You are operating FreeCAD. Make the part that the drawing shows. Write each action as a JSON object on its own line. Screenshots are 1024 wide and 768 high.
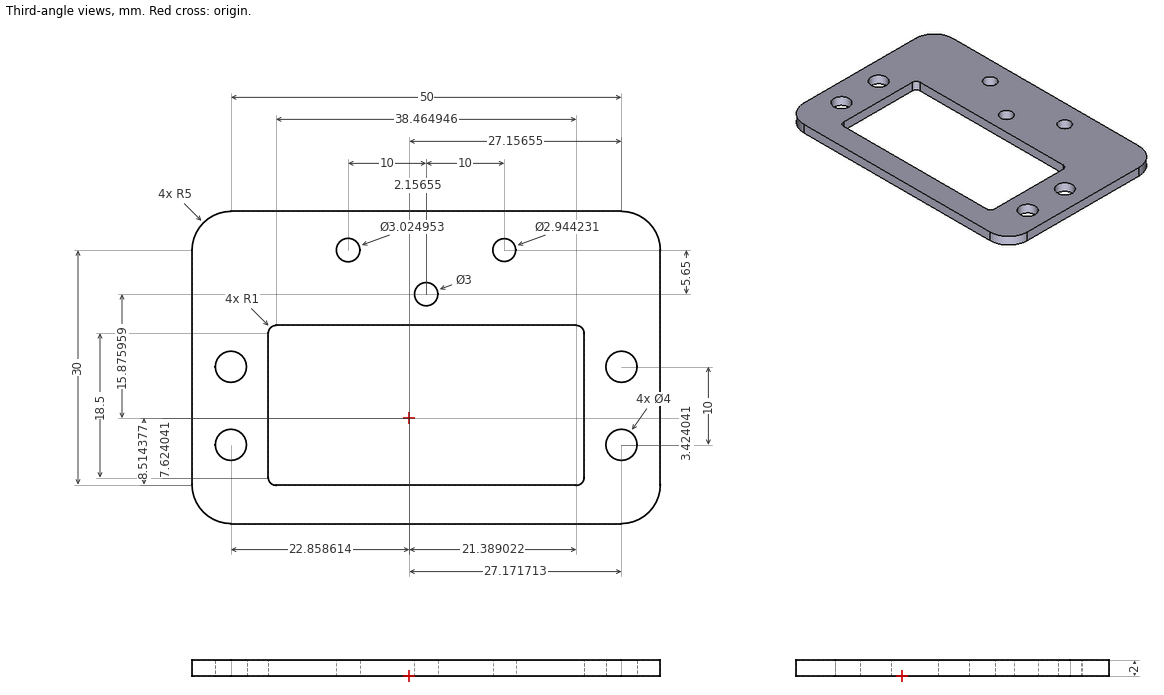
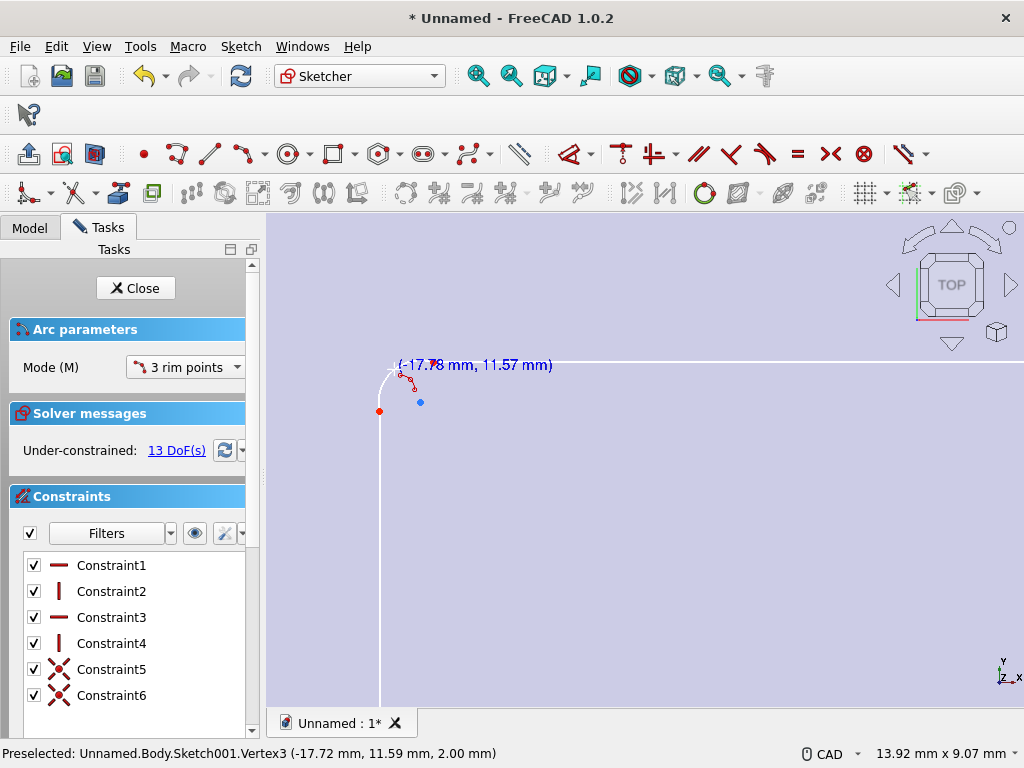
{"action": "scroll", "coordinate": [398, 371], "scroll_direction": "down", "scroll_amount": 9}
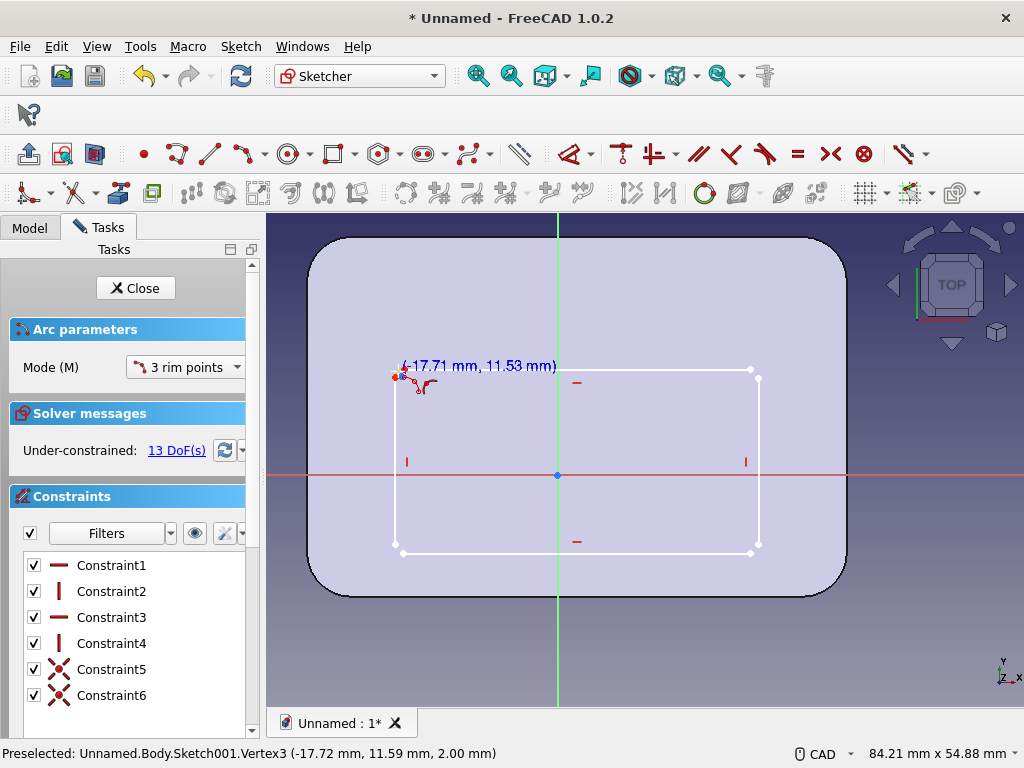
{"action": "scroll", "coordinate": [395, 544], "scroll_direction": "up", "scroll_amount": 2}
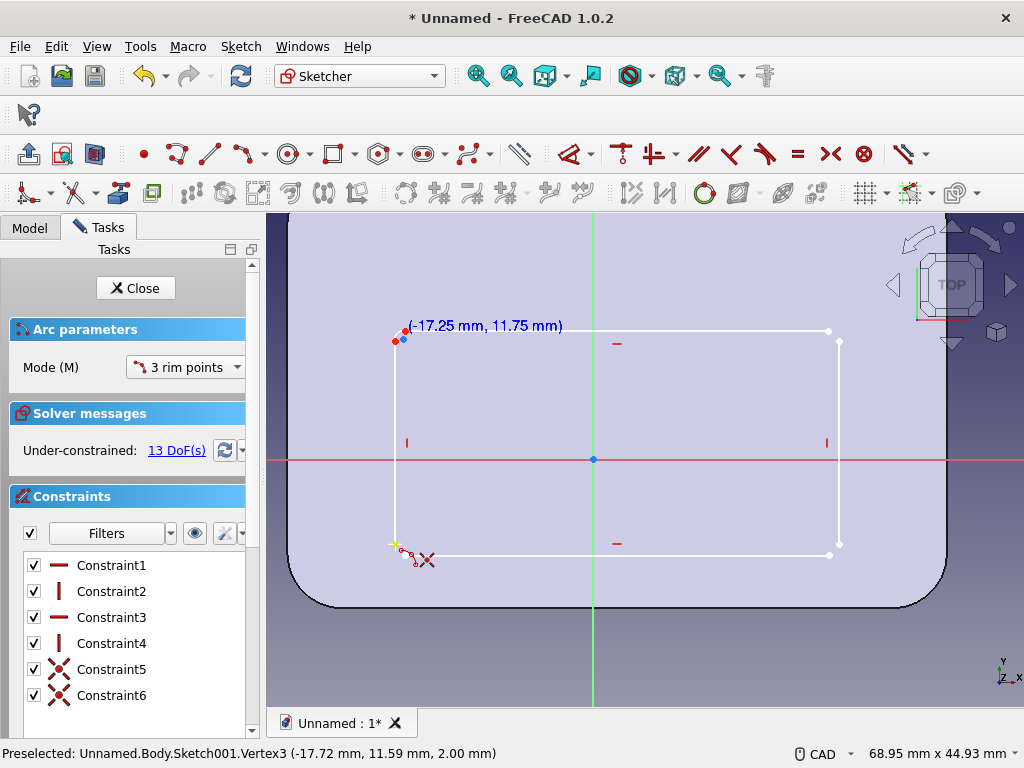
{"action": "left_click", "coordinate": [395, 545]}
{"action": "left_click", "coordinate": [408, 558]}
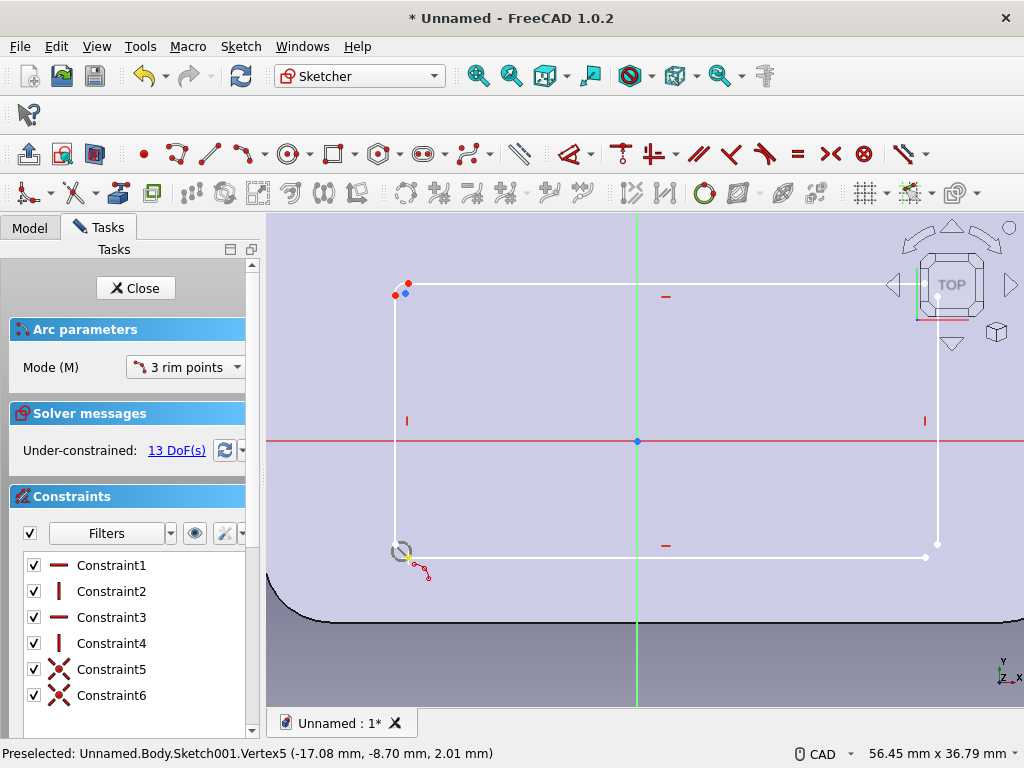
{"action": "scroll", "coordinate": [399, 553], "scroll_direction": "up", "scroll_amount": 7}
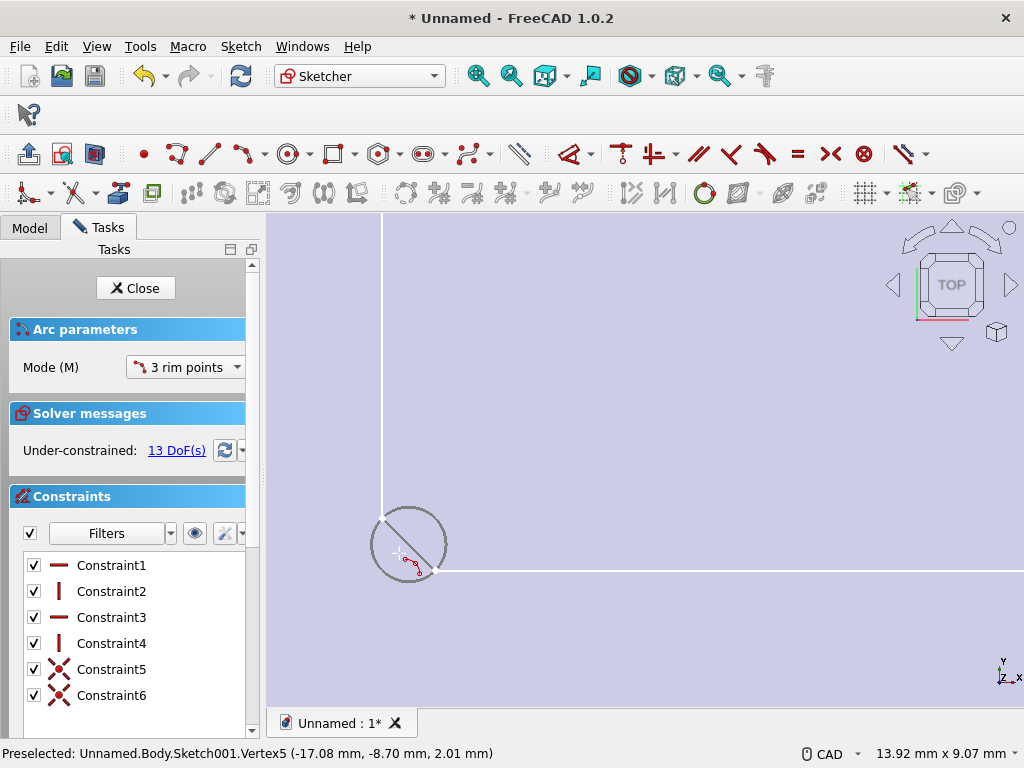
{"action": "left_click", "coordinate": [397, 551]}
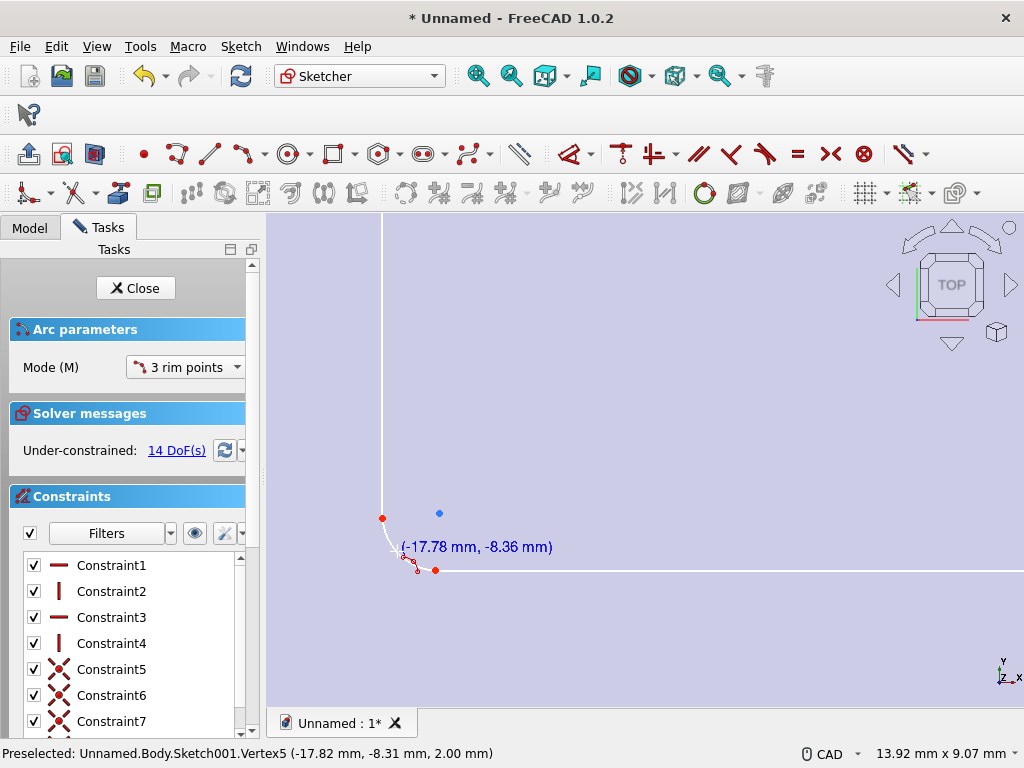
{"action": "scroll", "coordinate": [397, 549], "scroll_direction": "down", "scroll_amount": 9}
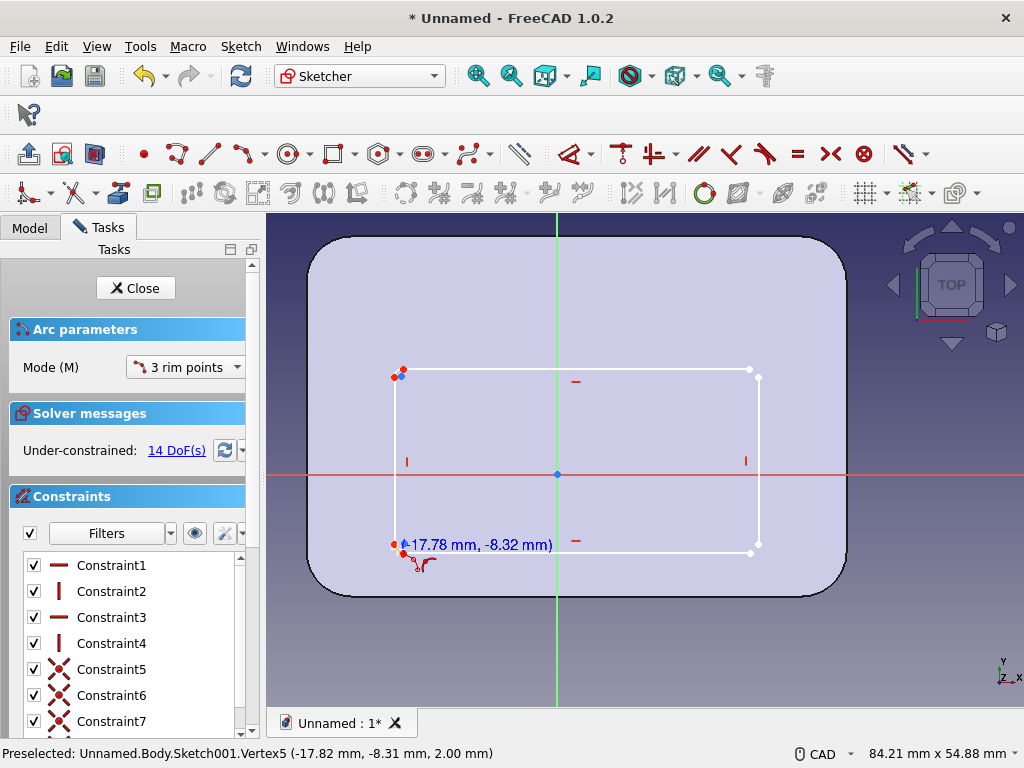
{"action": "scroll", "coordinate": [750, 552], "scroll_direction": "up", "scroll_amount": 2}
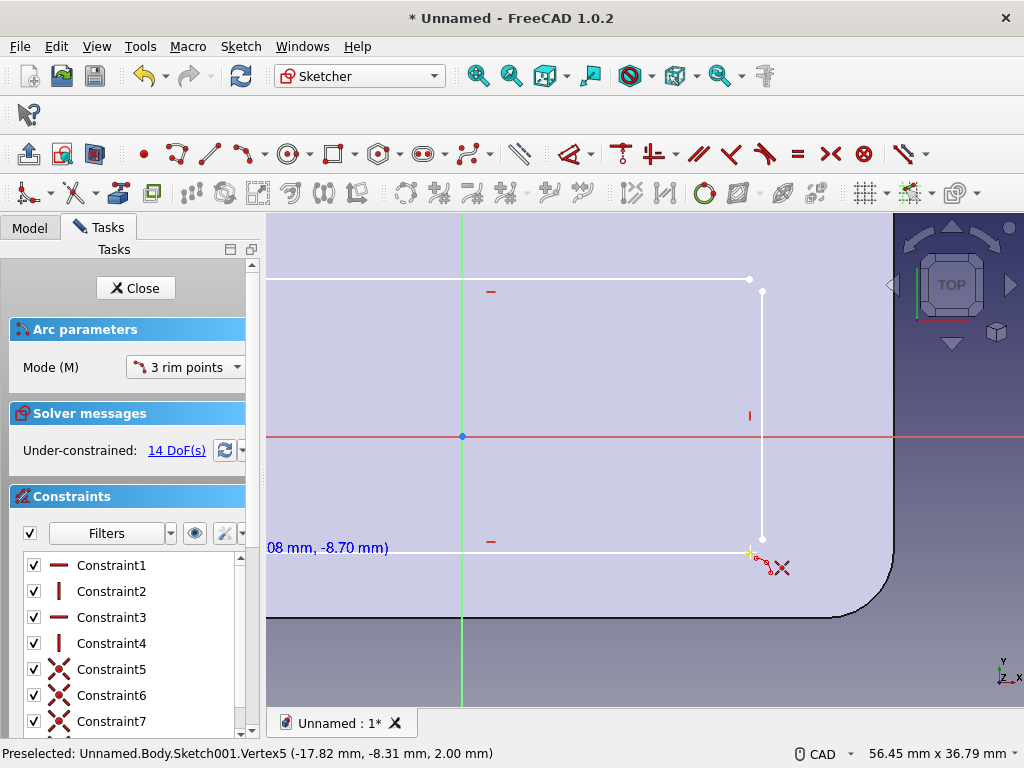
{"action": "left_click", "coordinate": [750, 553]}
{"action": "left_click", "coordinate": [762, 540]}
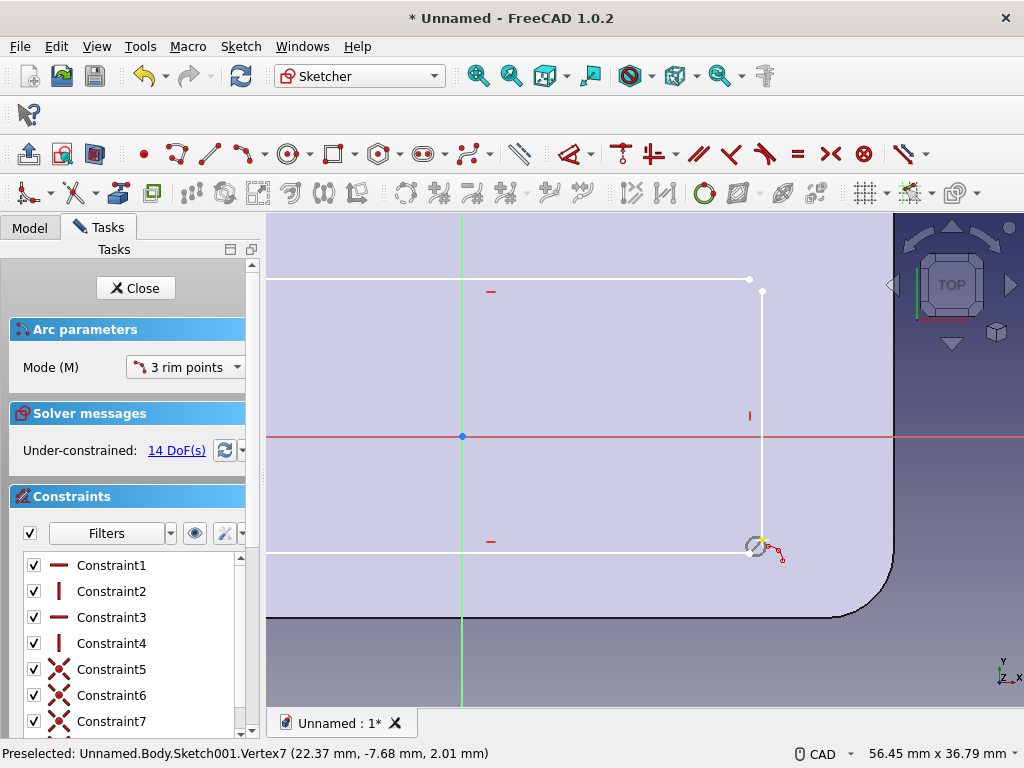
{"action": "scroll", "coordinate": [759, 548], "scroll_direction": "up", "scroll_amount": 7}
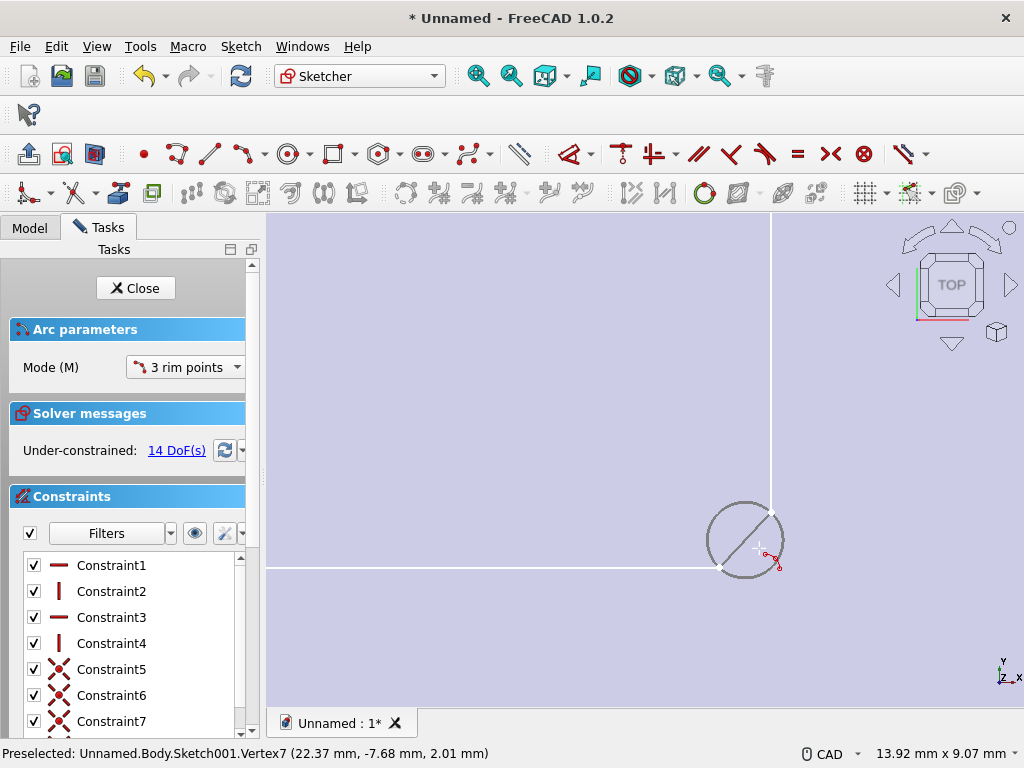
{"action": "left_click", "coordinate": [756, 548]}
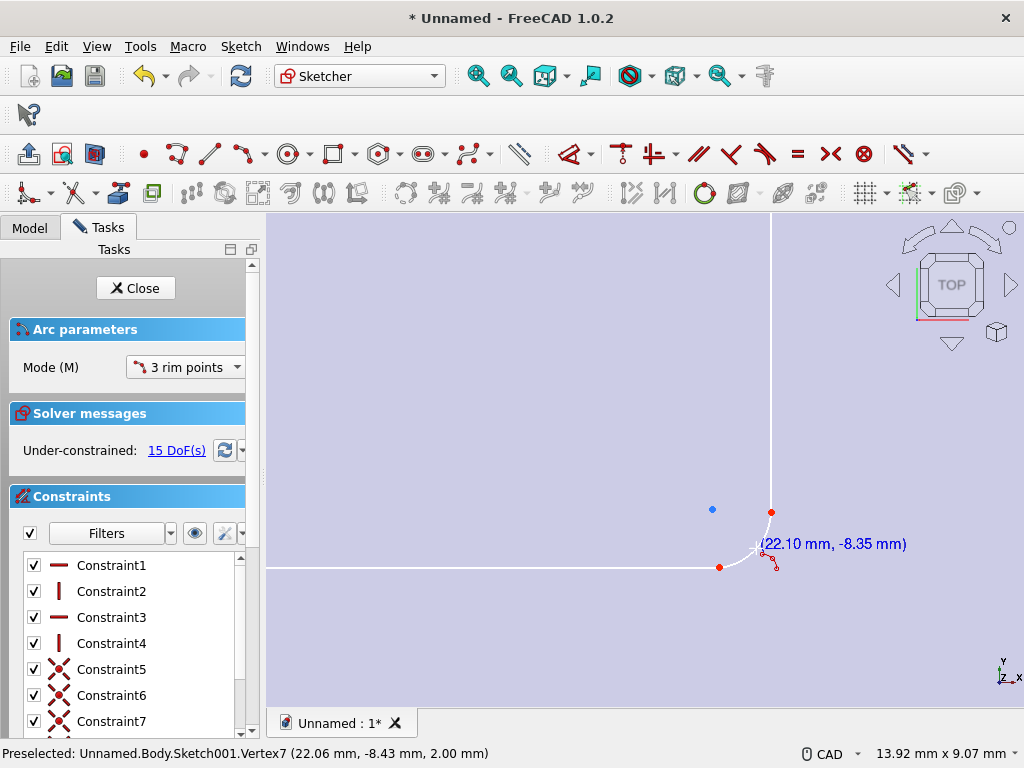
{"action": "scroll", "coordinate": [756, 550], "scroll_direction": "down", "scroll_amount": 9}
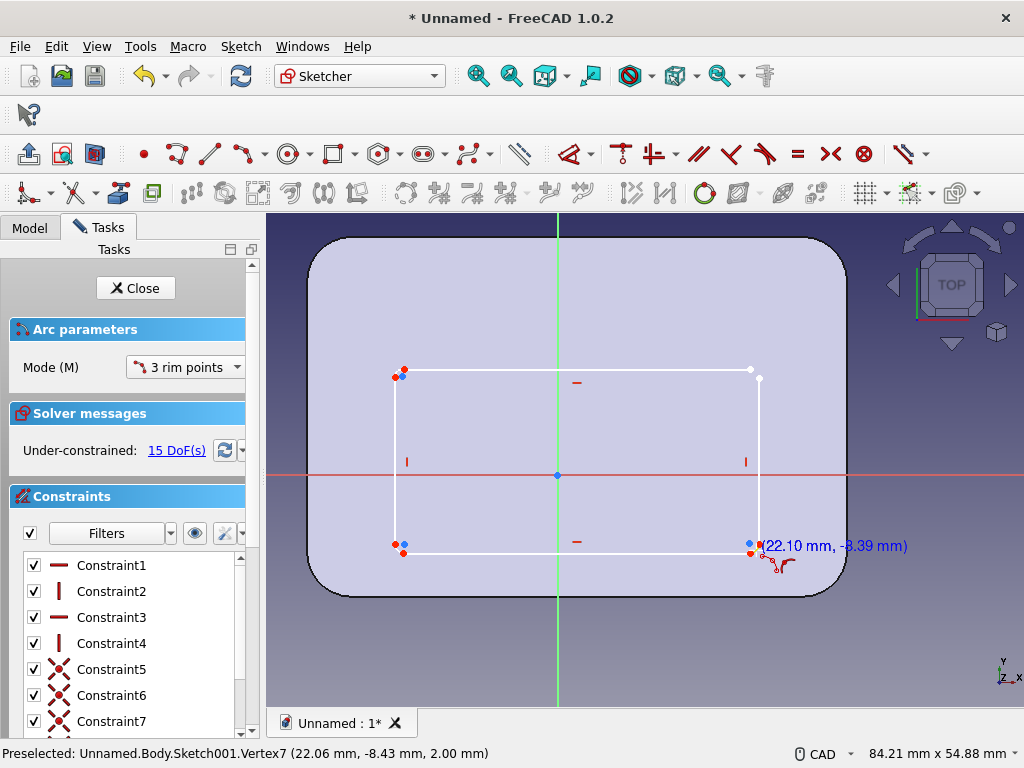
{"action": "scroll", "coordinate": [759, 377], "scroll_direction": "up", "scroll_amount": 2}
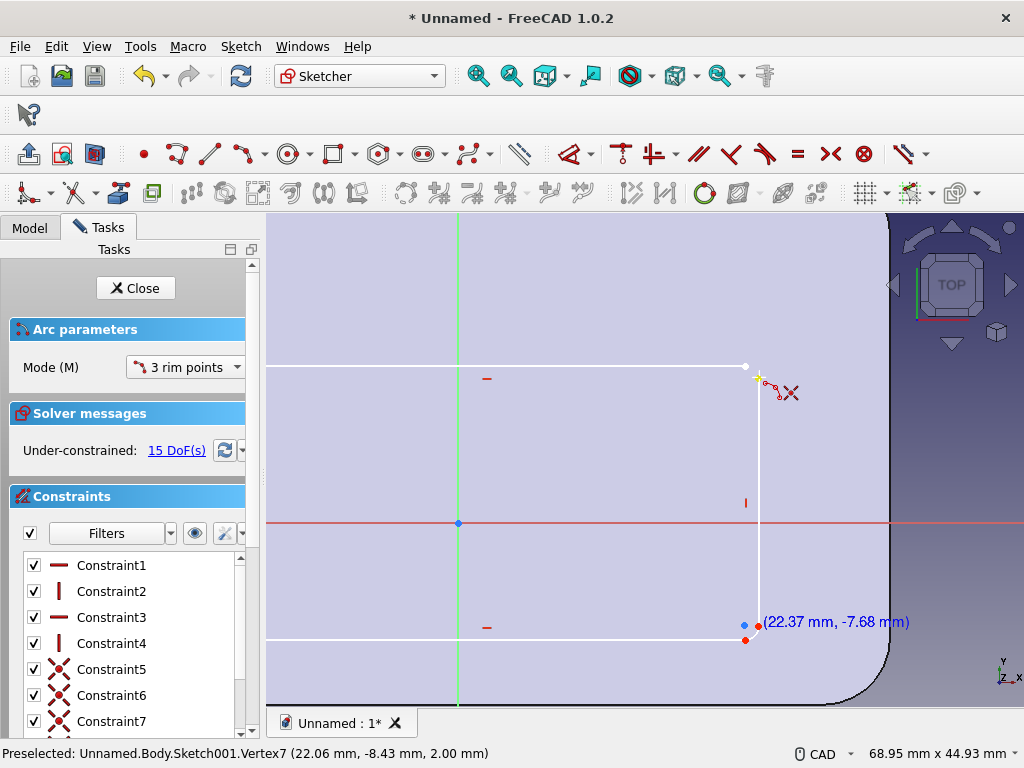
{"action": "left_click", "coordinate": [759, 379]}
{"action": "left_click", "coordinate": [745, 366]}